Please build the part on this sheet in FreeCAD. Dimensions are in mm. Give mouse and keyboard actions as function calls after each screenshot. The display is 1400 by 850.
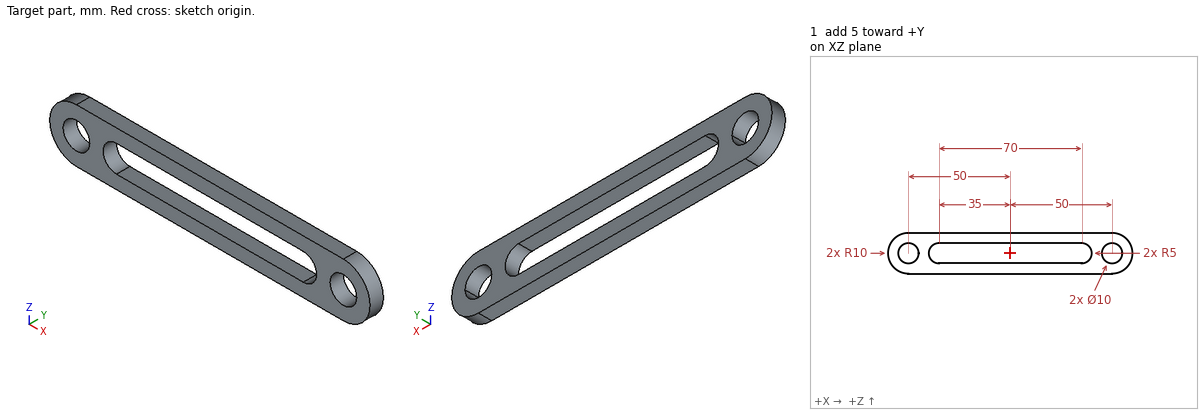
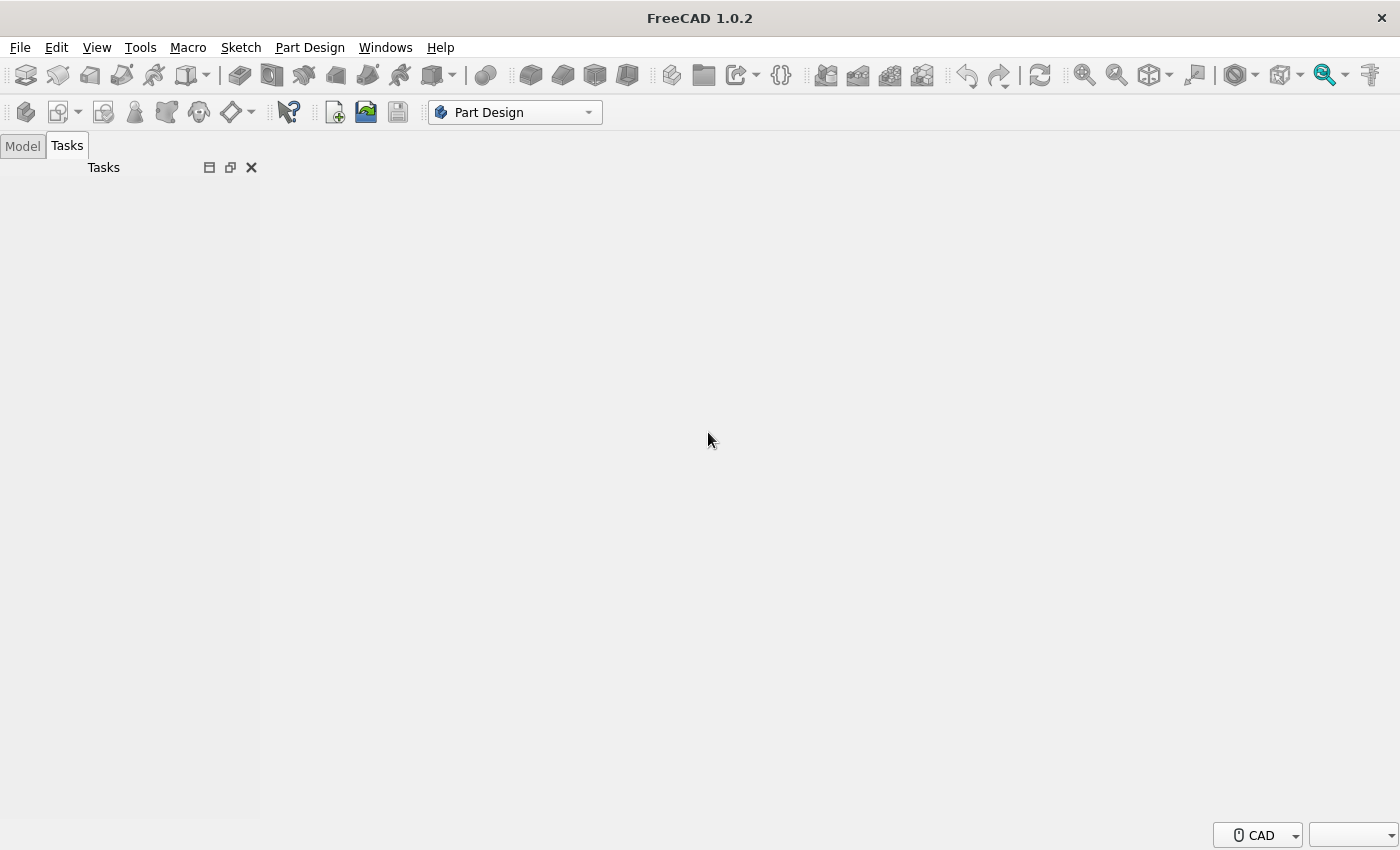
click(334, 112)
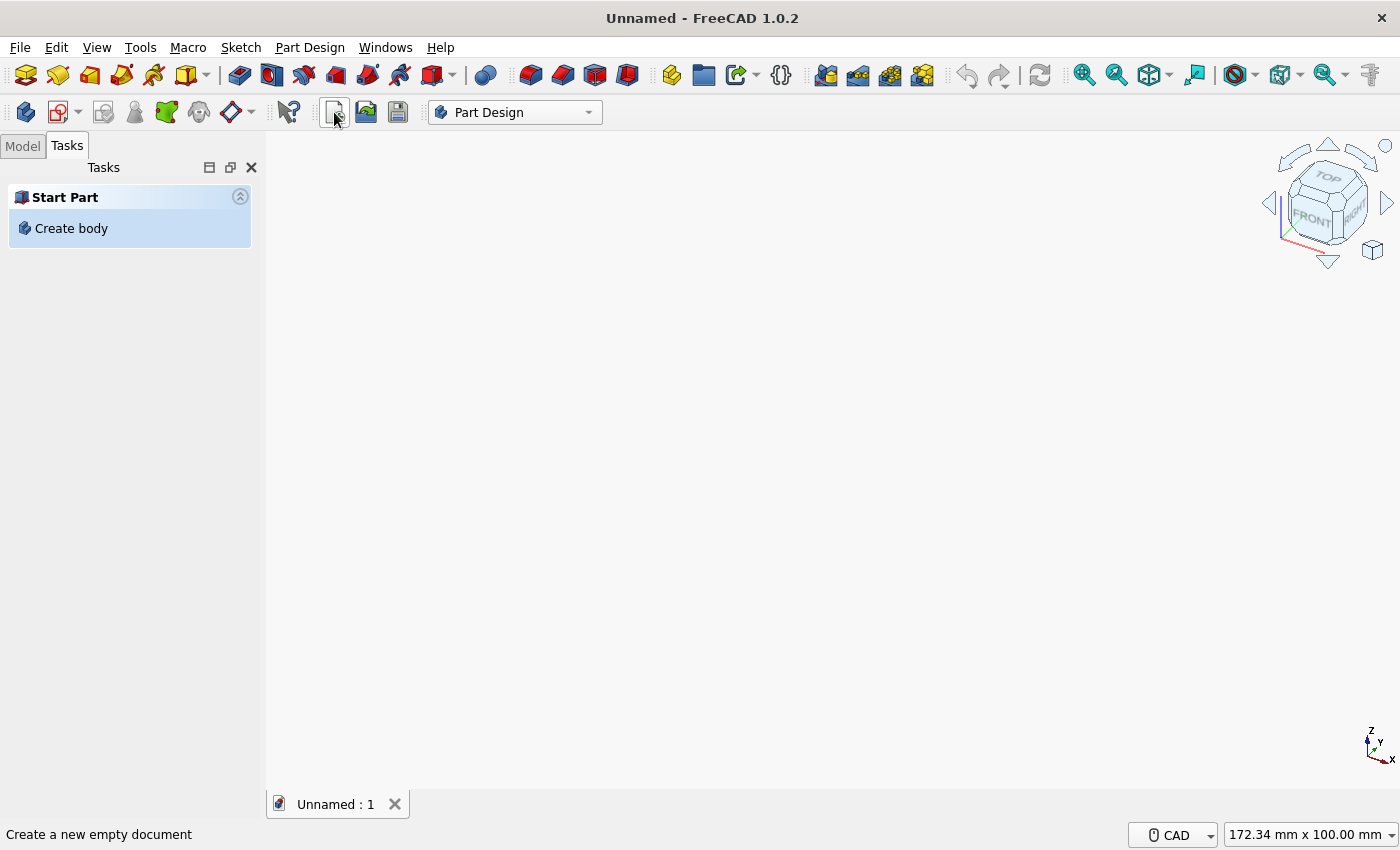
click(58, 112)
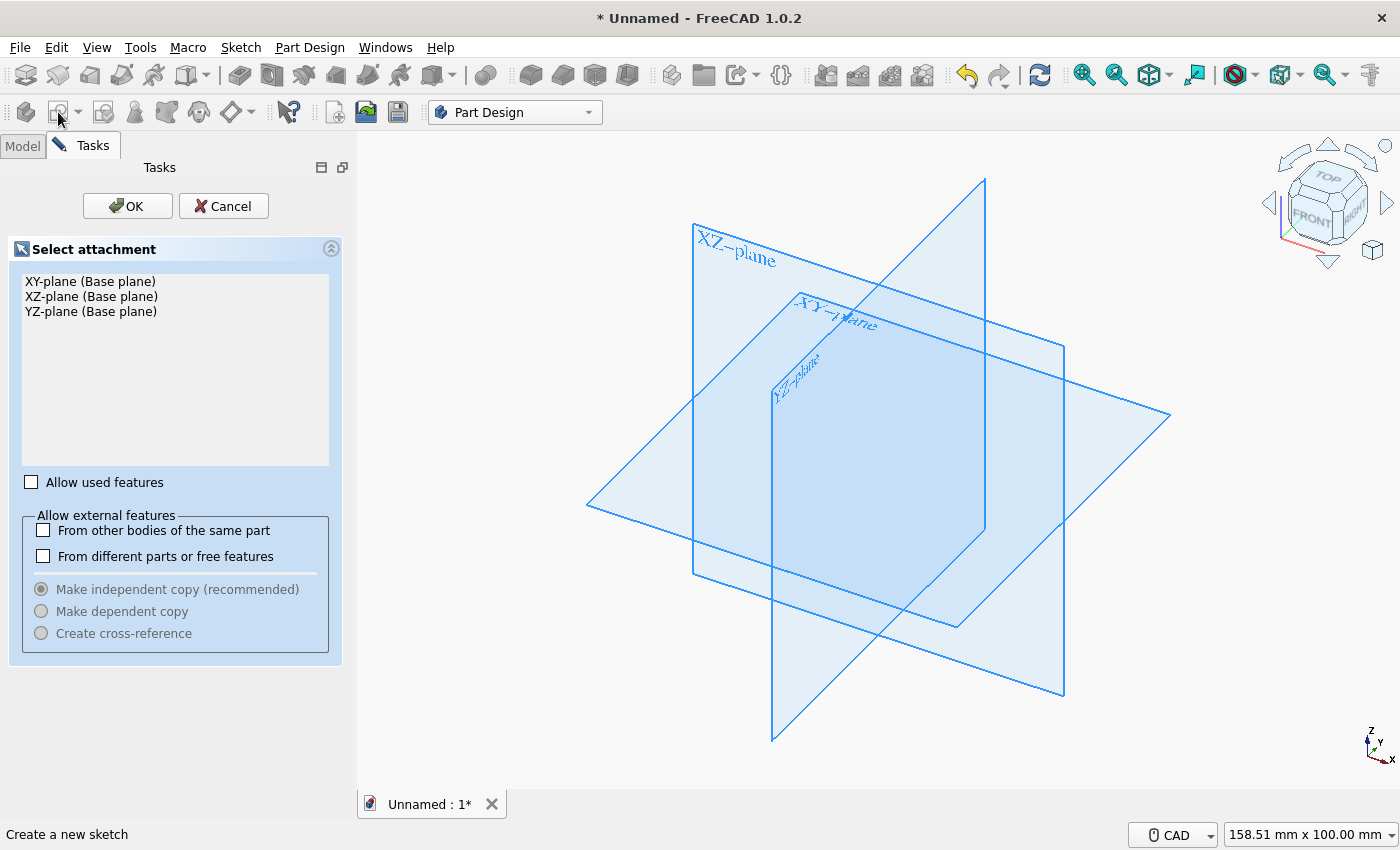
click(82, 296)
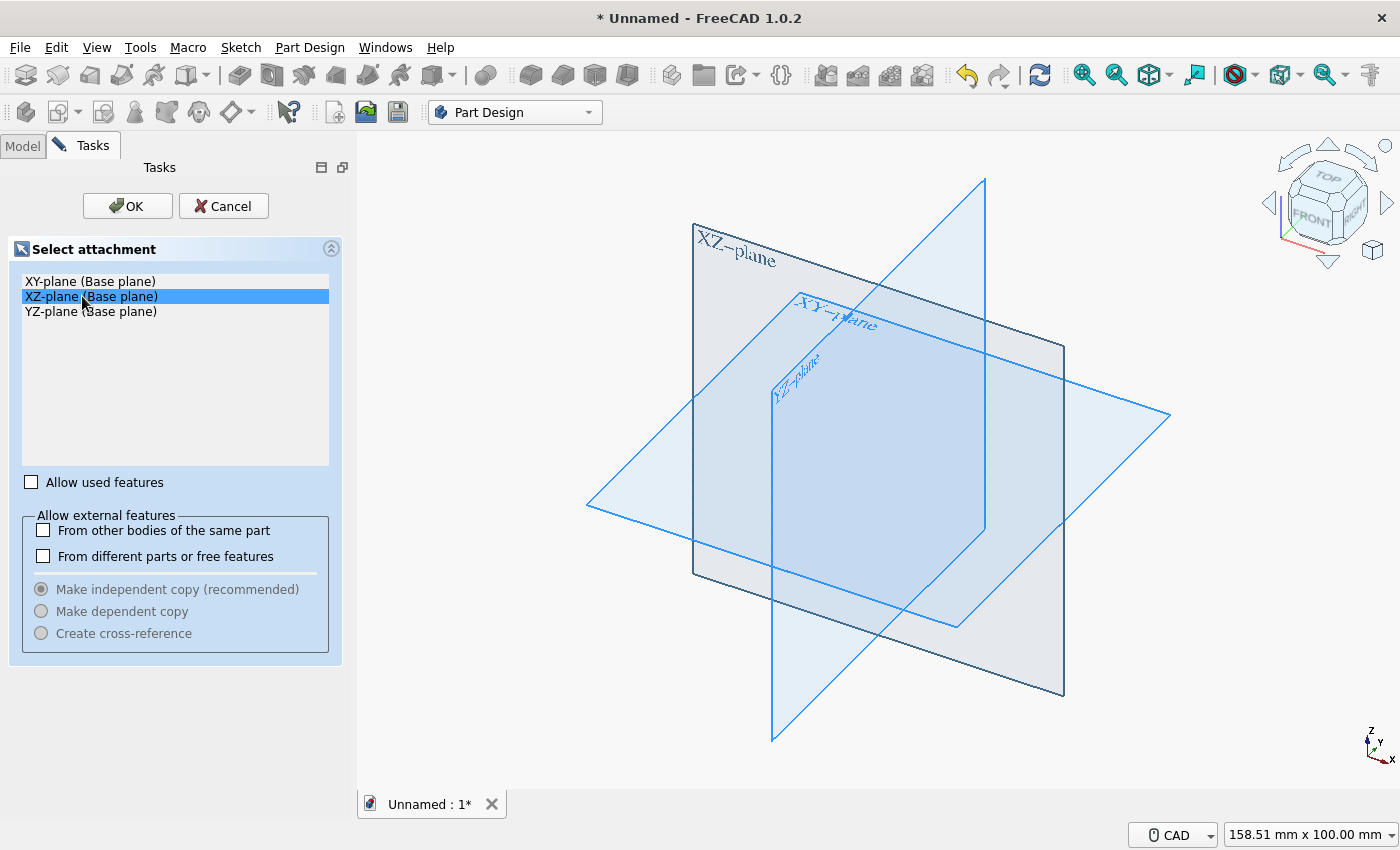
click(128, 206)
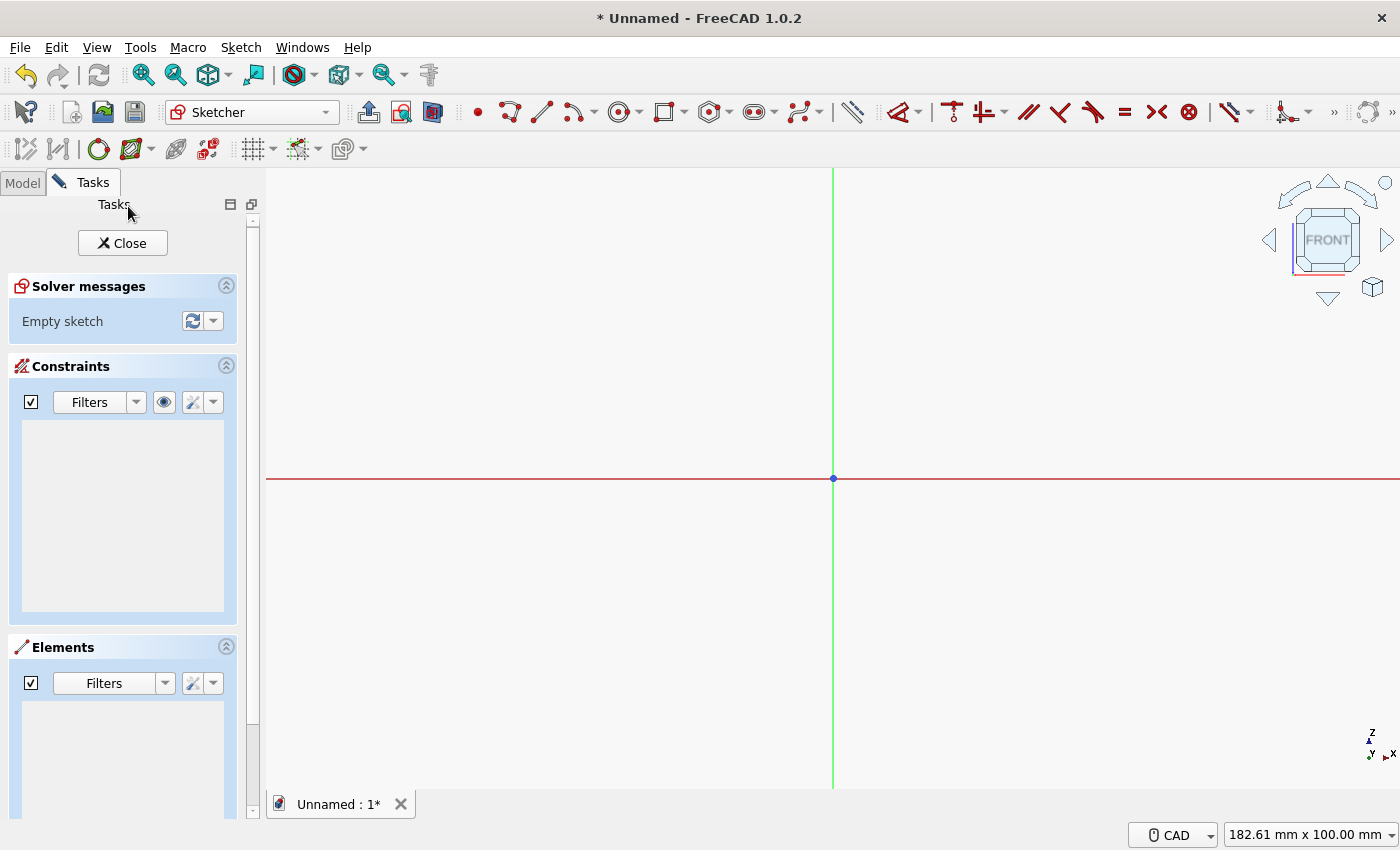
key(g)
key(s)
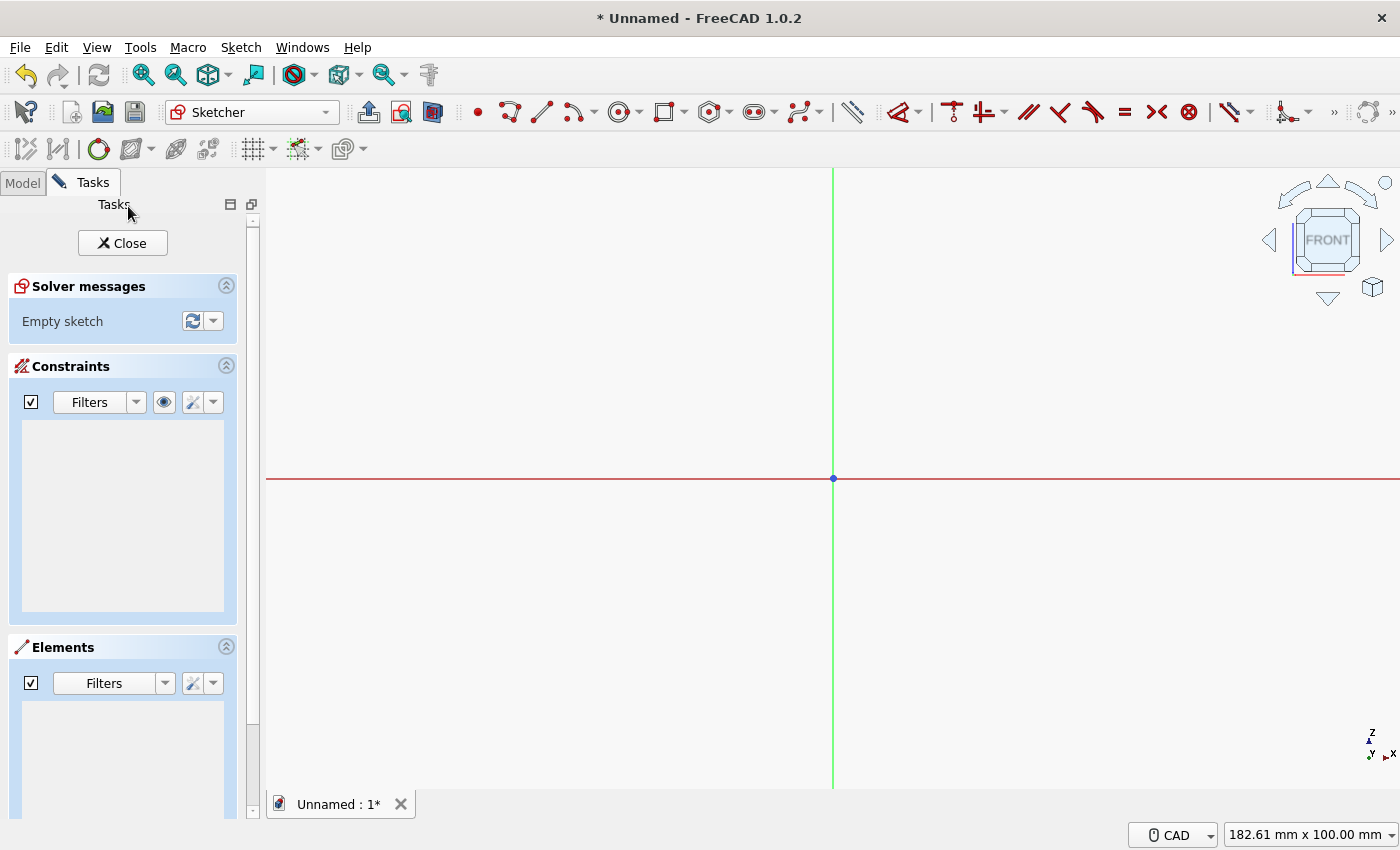
click(523, 478)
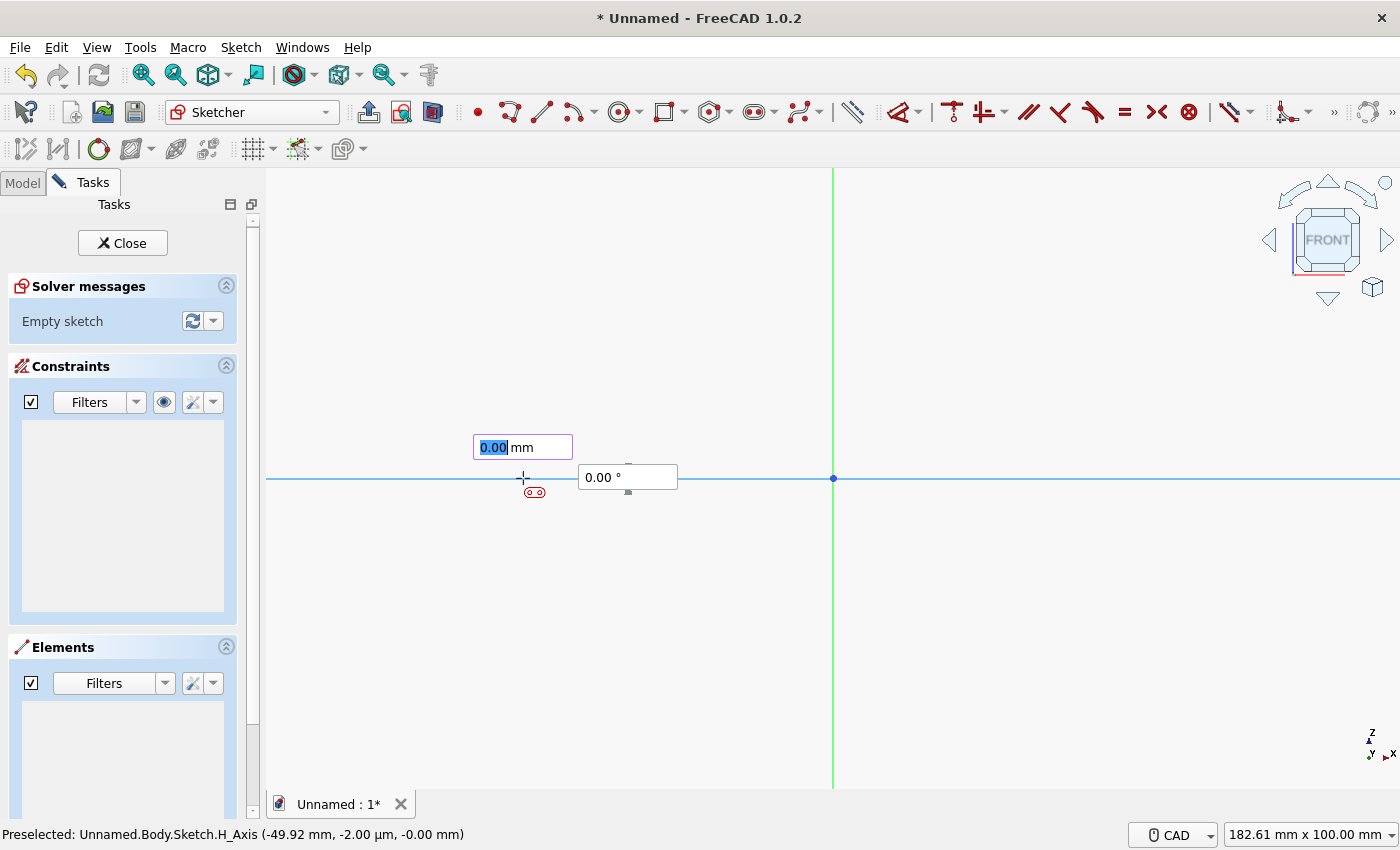
click(1144, 470)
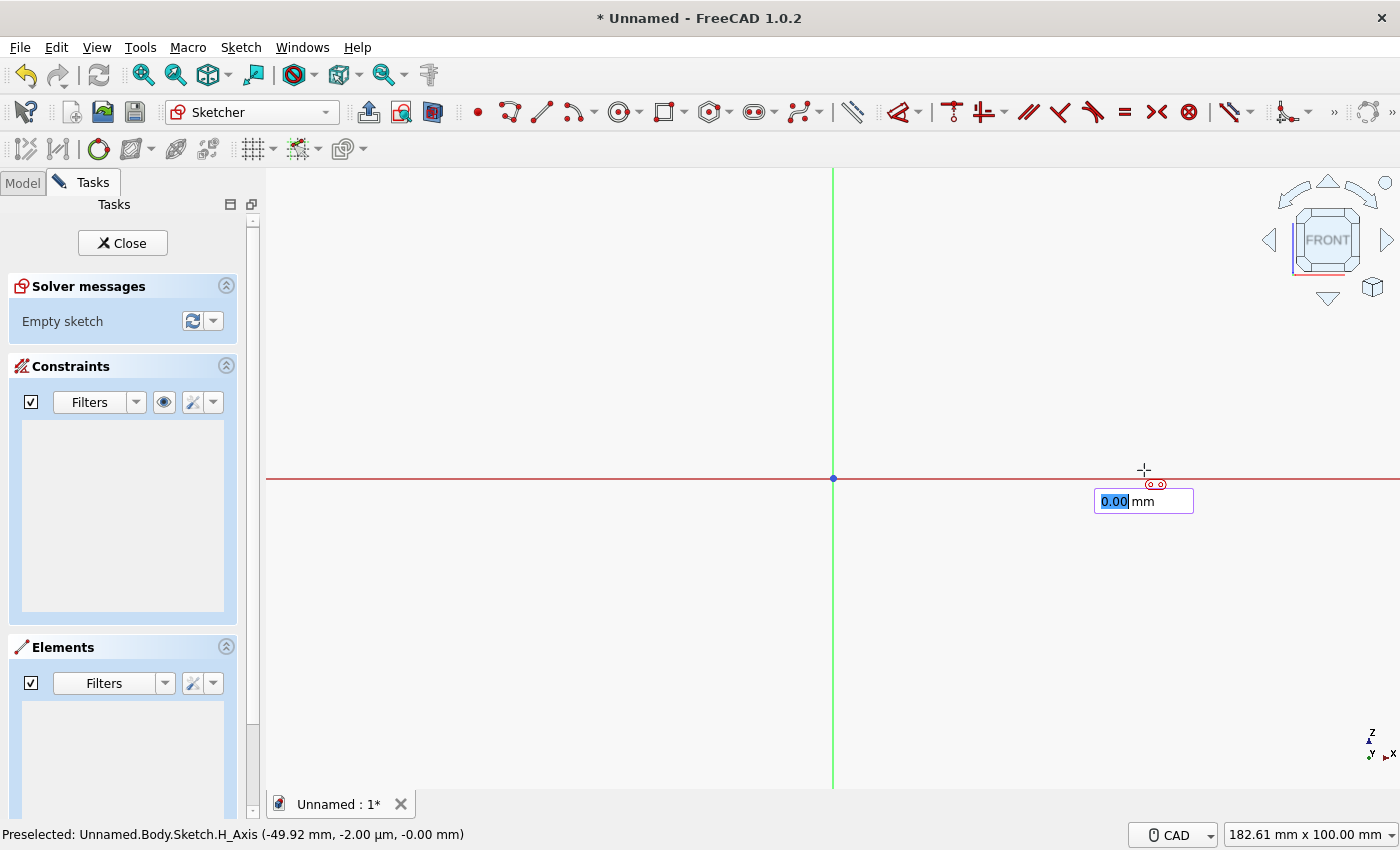
click(926, 541)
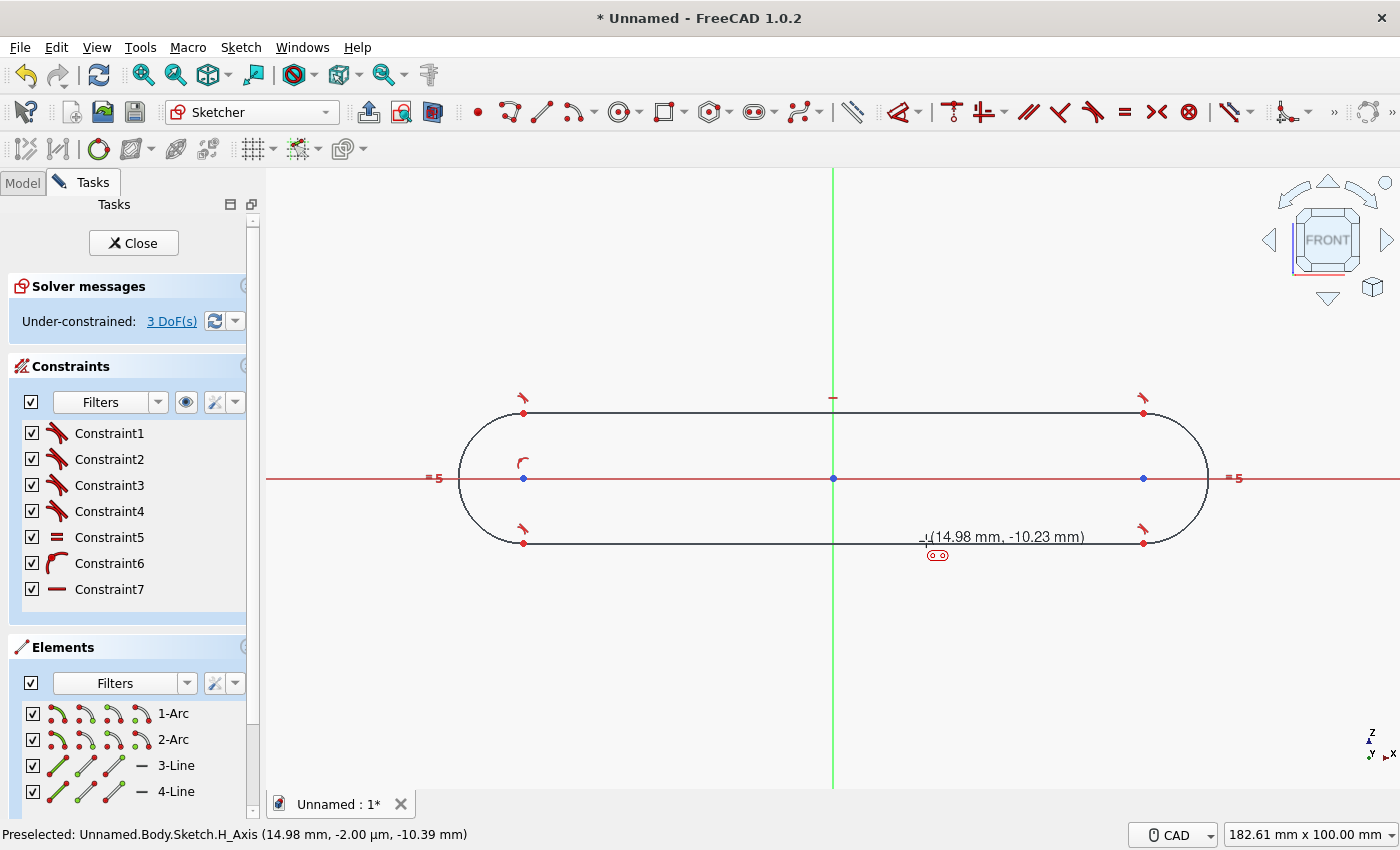
click(616, 478)